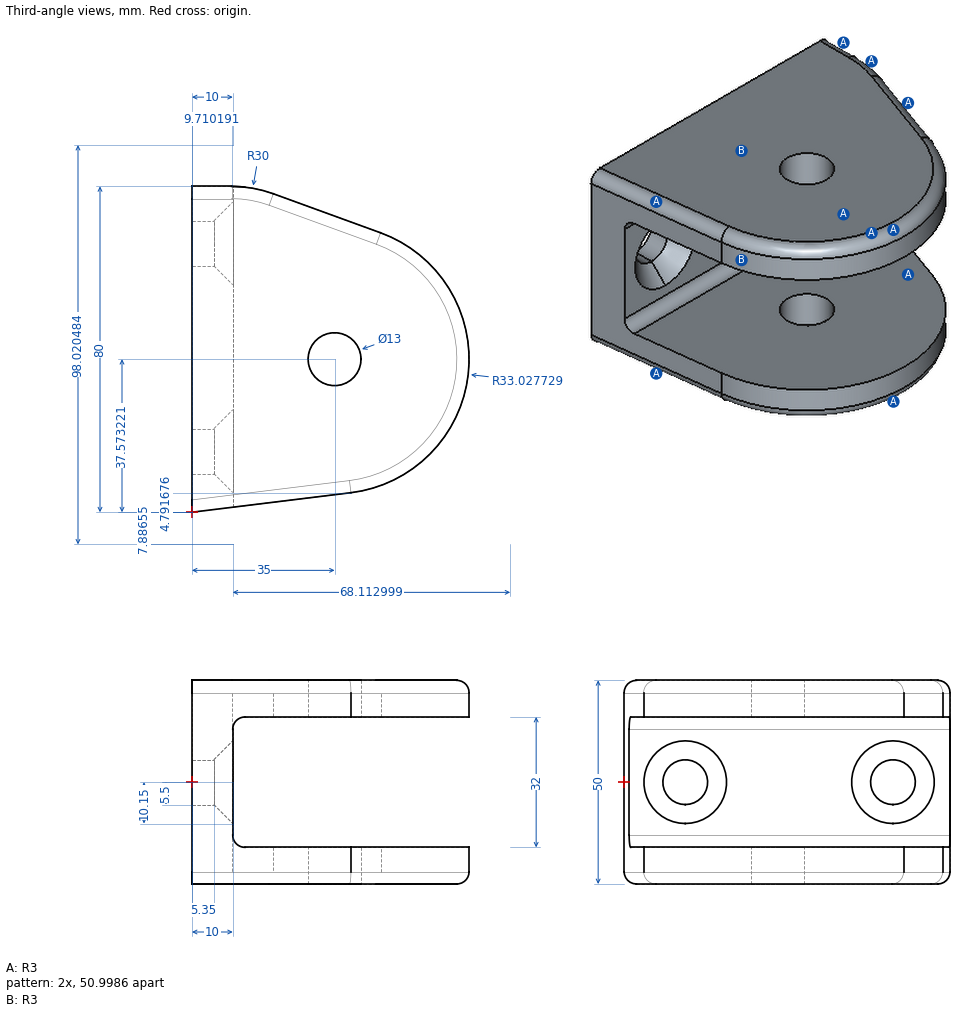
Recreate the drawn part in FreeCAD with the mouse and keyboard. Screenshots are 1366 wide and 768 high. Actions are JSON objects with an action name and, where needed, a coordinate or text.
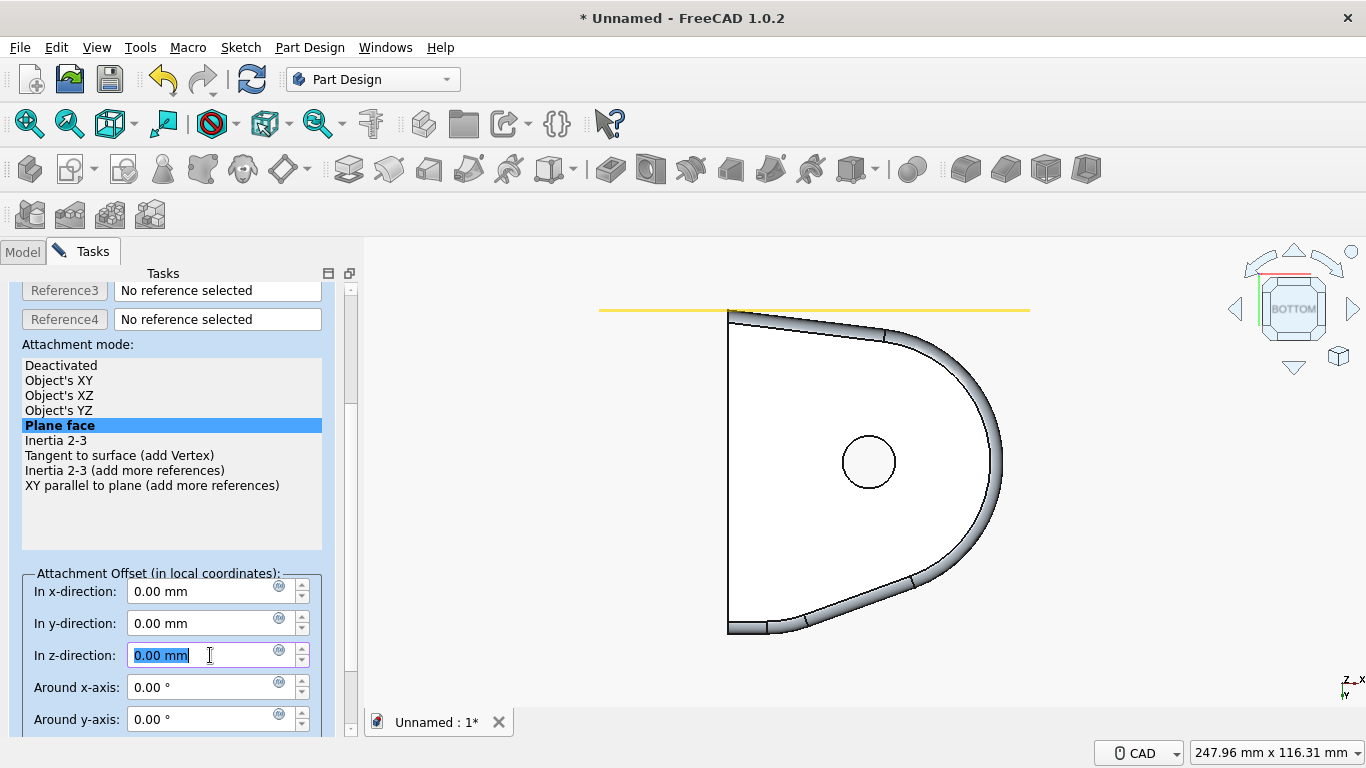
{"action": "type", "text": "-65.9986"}
{"action": "key", "text": "Tab"}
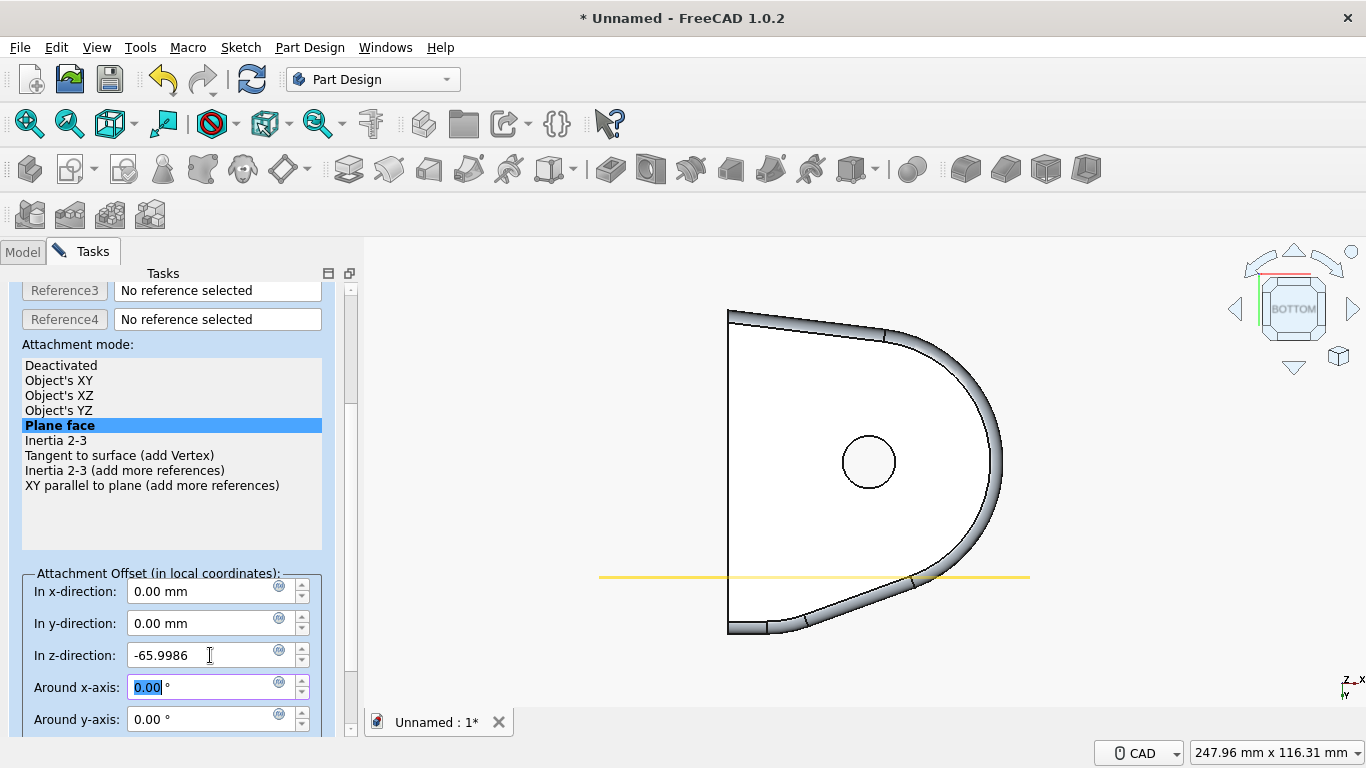
{"action": "scroll", "coordinate": [351, 510], "scroll_direction": "up", "scroll_amount": 4}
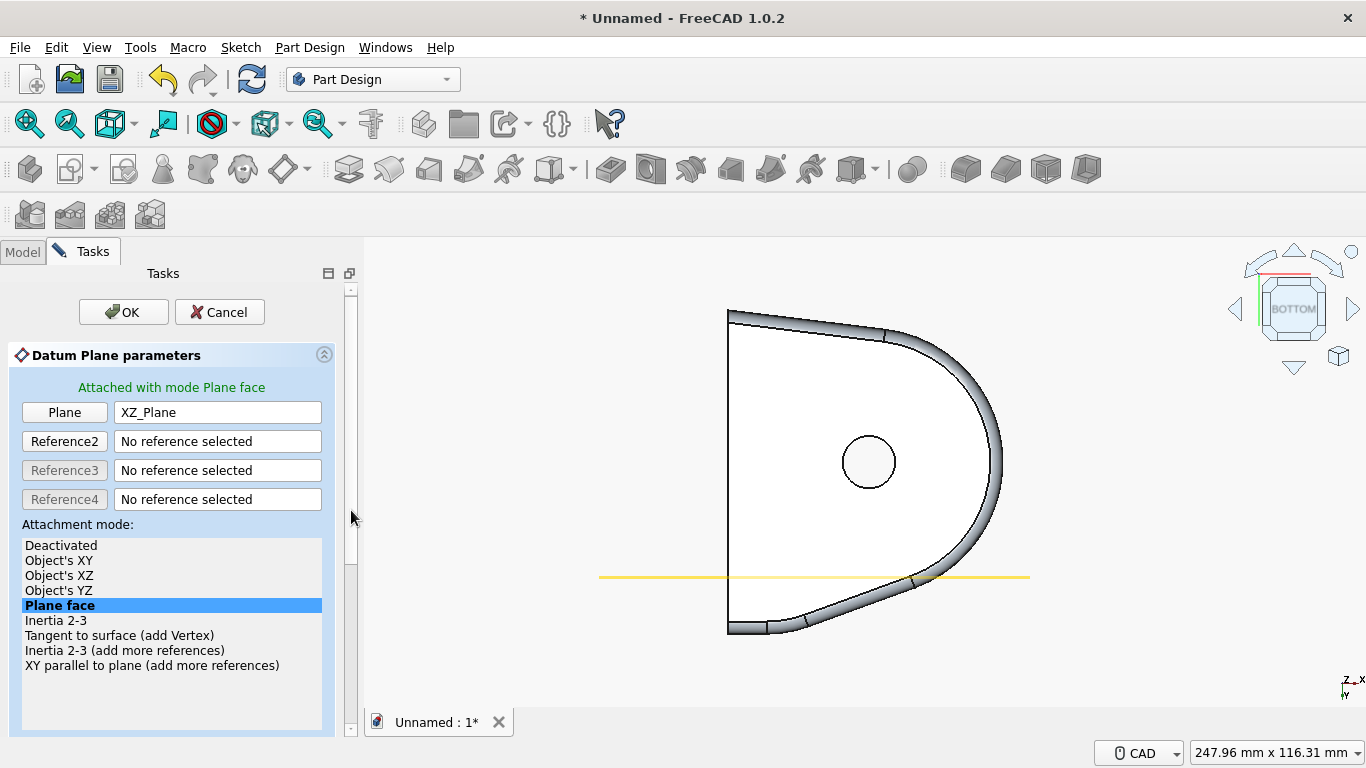
{"action": "left_click", "coordinate": [124, 312]}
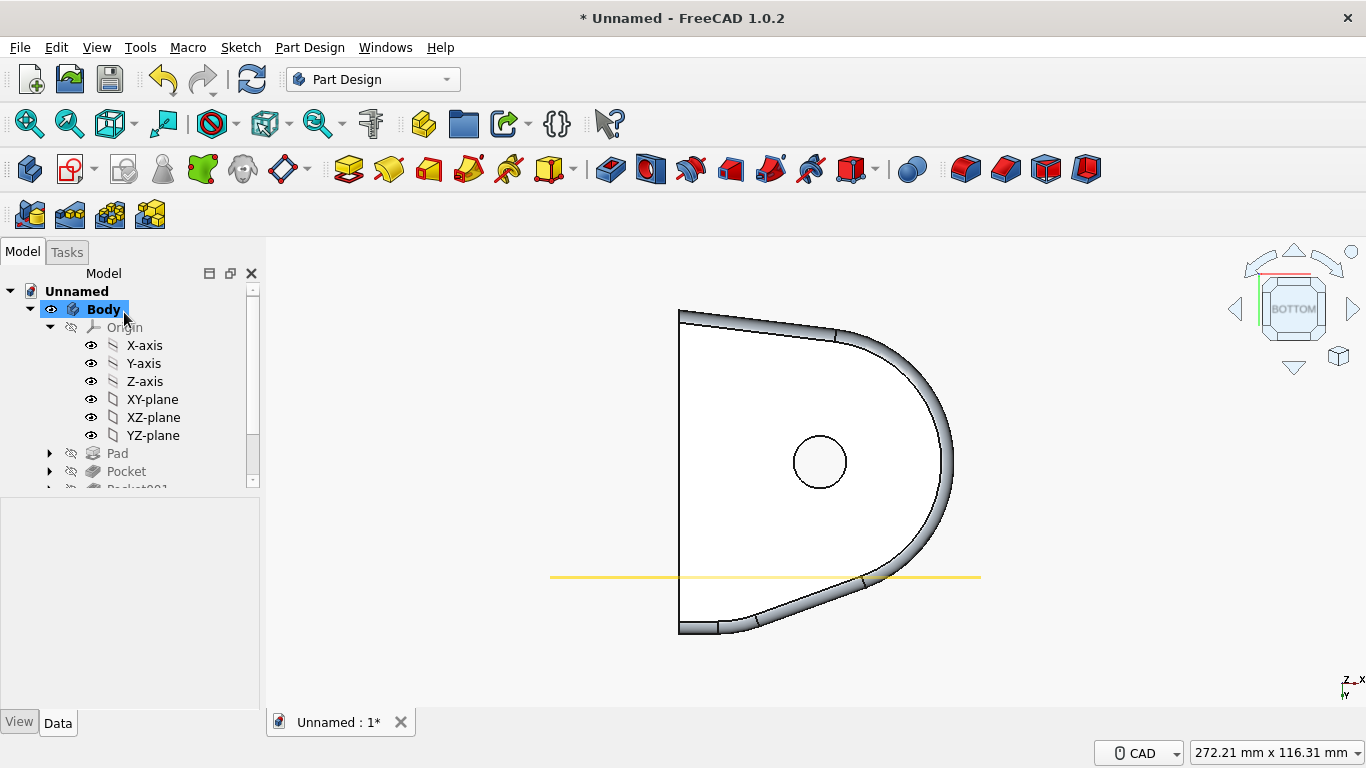
{"action": "scroll", "coordinate": [100, 377], "scroll_direction": "down", "scroll_amount": 3}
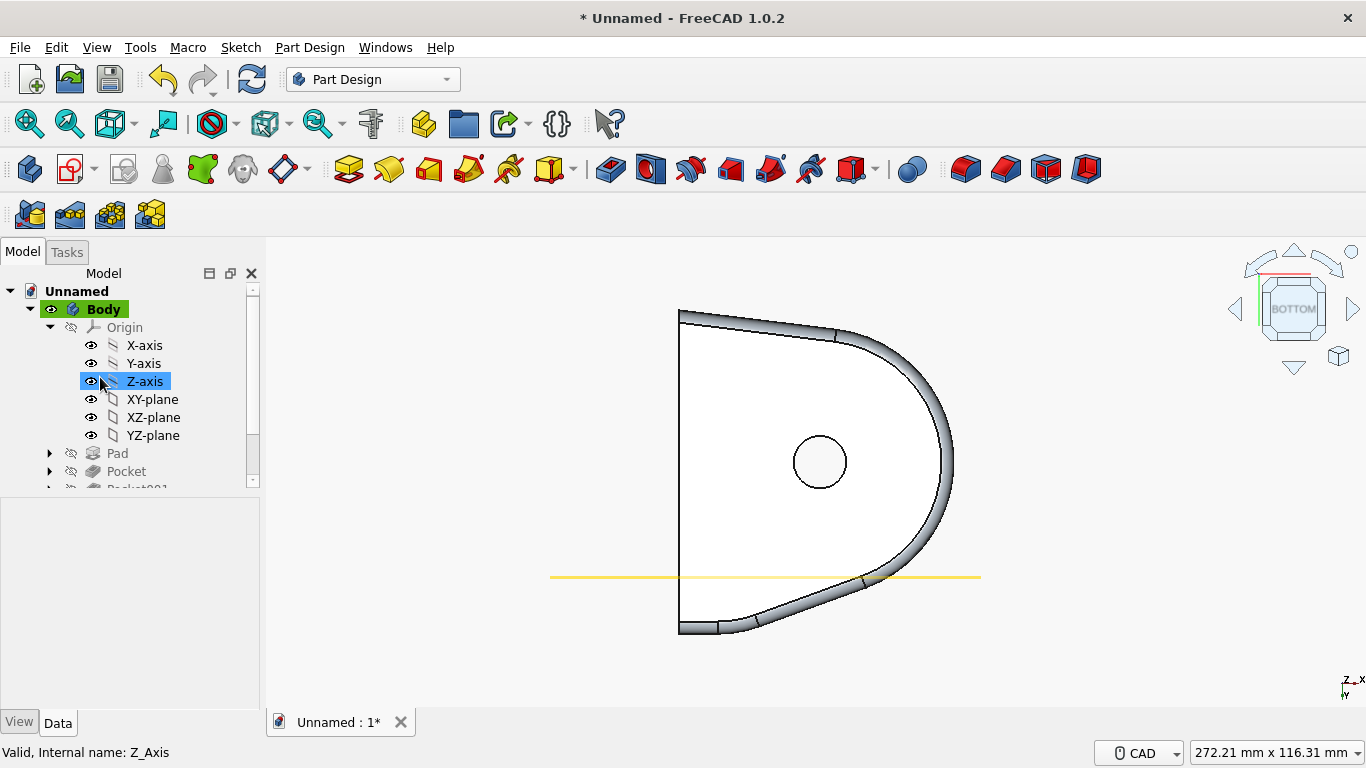
{"action": "left_click", "coordinate": [116, 471]}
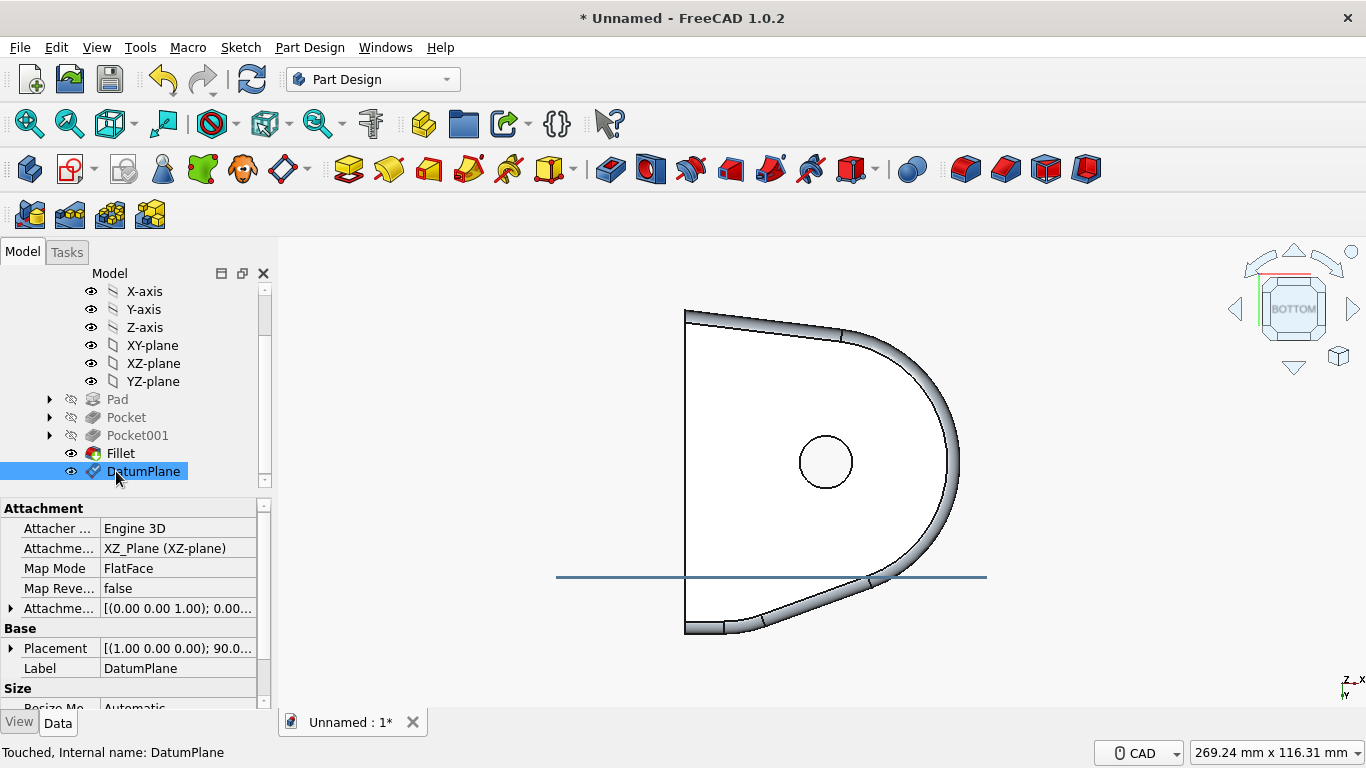
{"action": "left_click", "coordinate": [70, 170]}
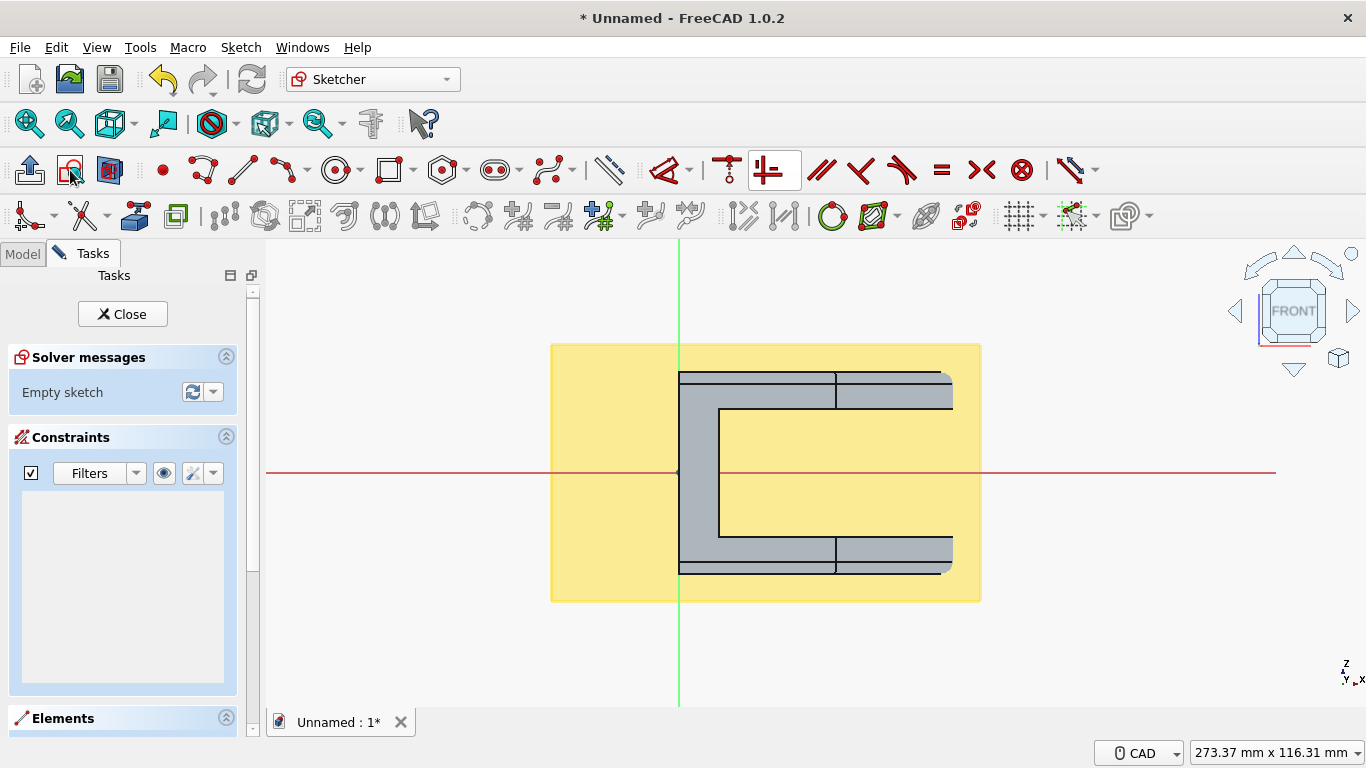
{"action": "left_click", "coordinate": [110, 170]}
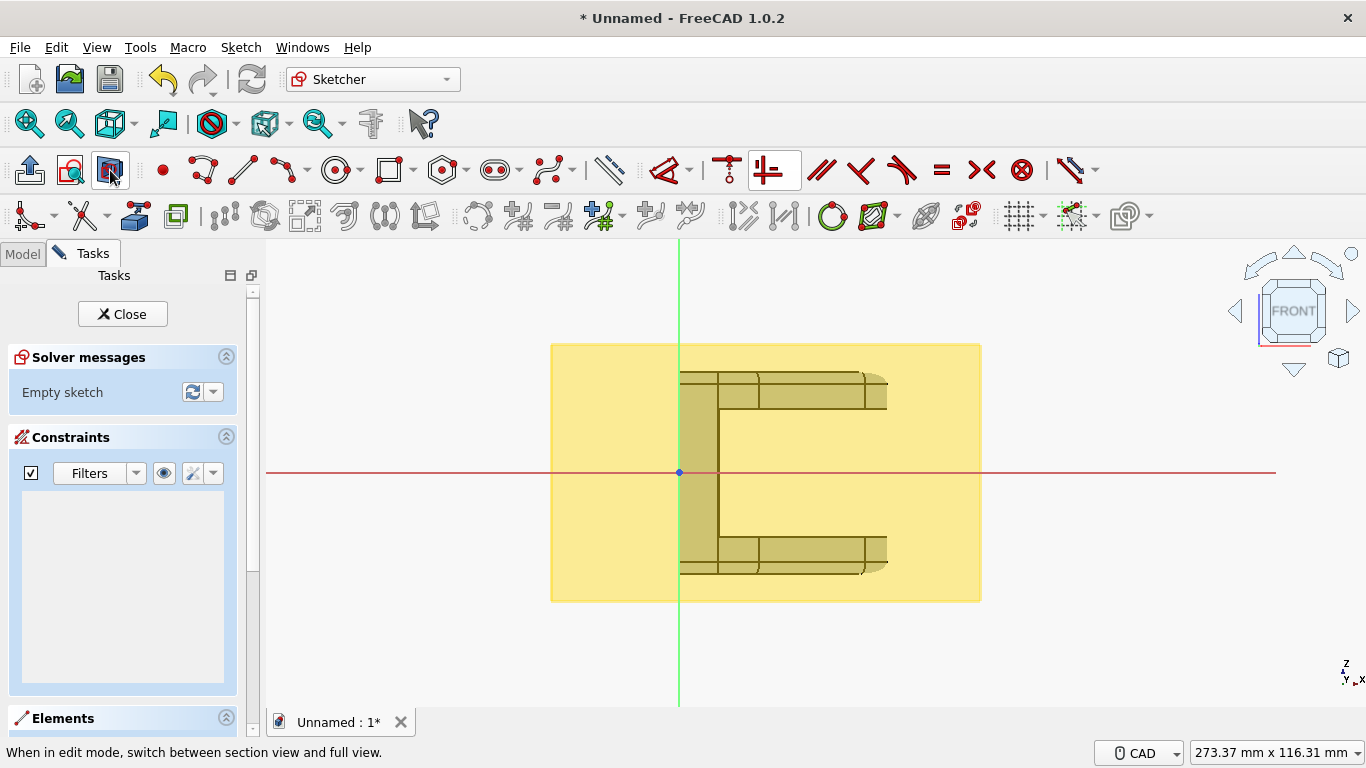
{"action": "scroll", "coordinate": [692, 497], "scroll_direction": "up", "scroll_amount": 10}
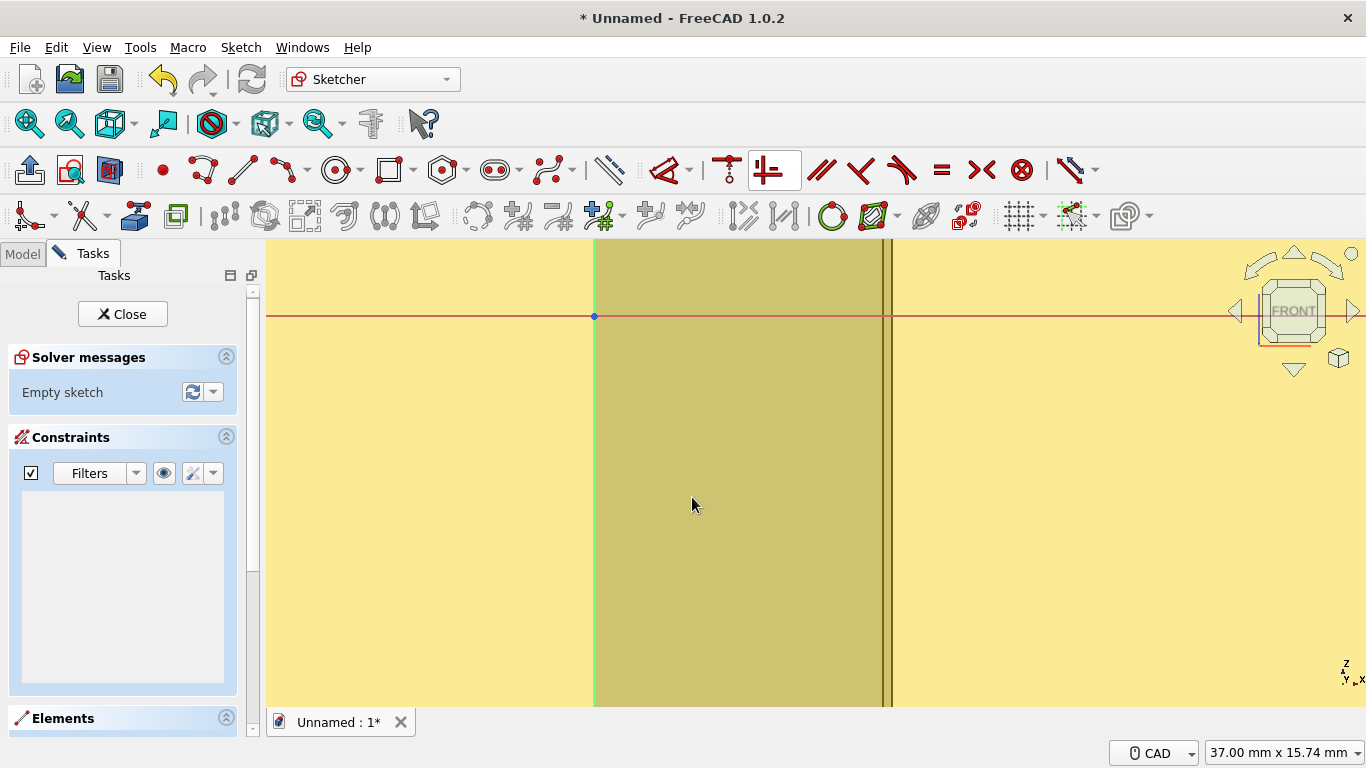
{"action": "left_click", "coordinate": [204, 170]}